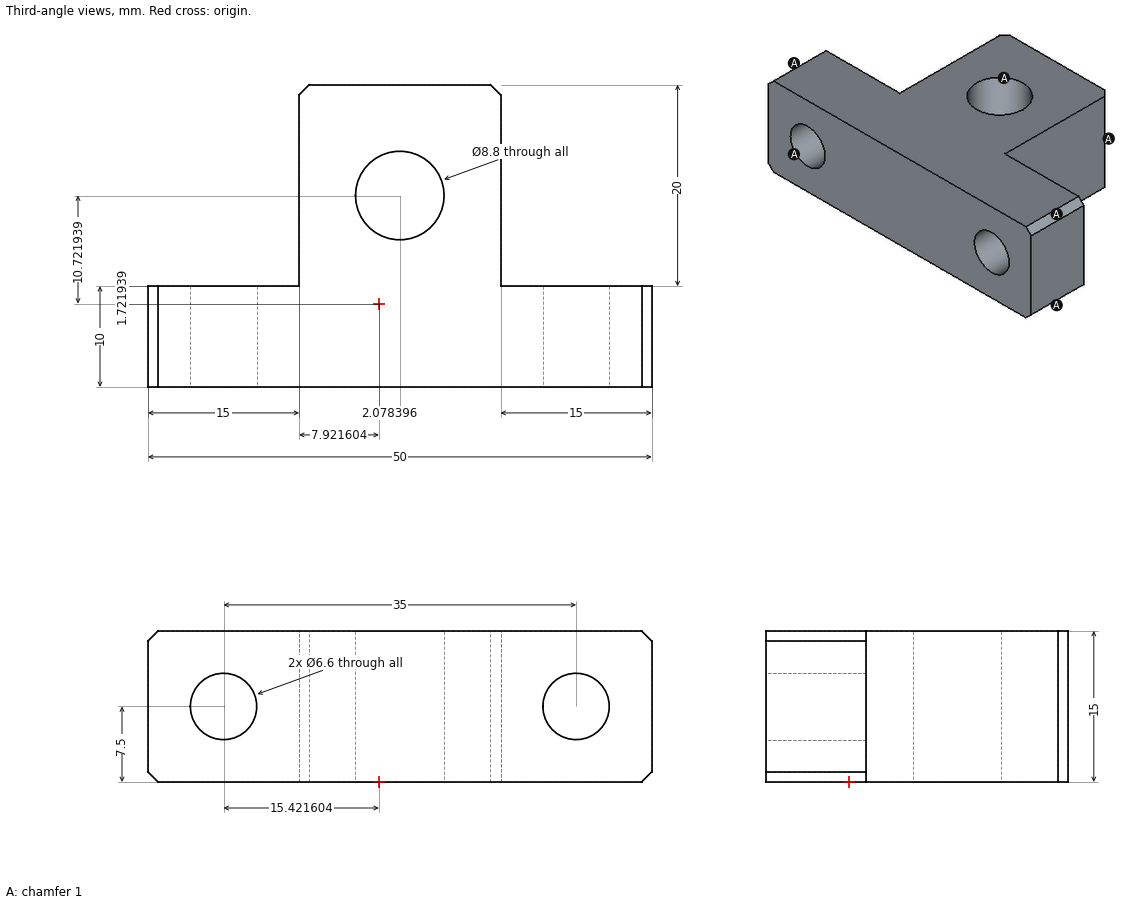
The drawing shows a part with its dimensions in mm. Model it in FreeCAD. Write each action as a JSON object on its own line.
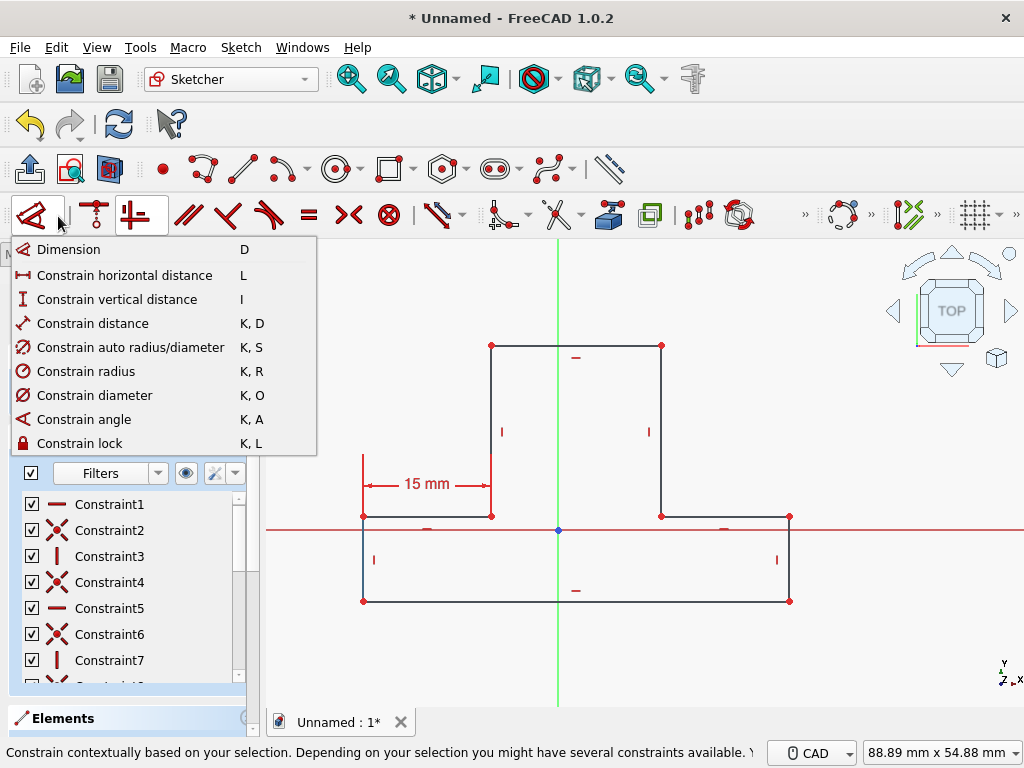
{"action": "left_click", "coordinate": [164, 299]}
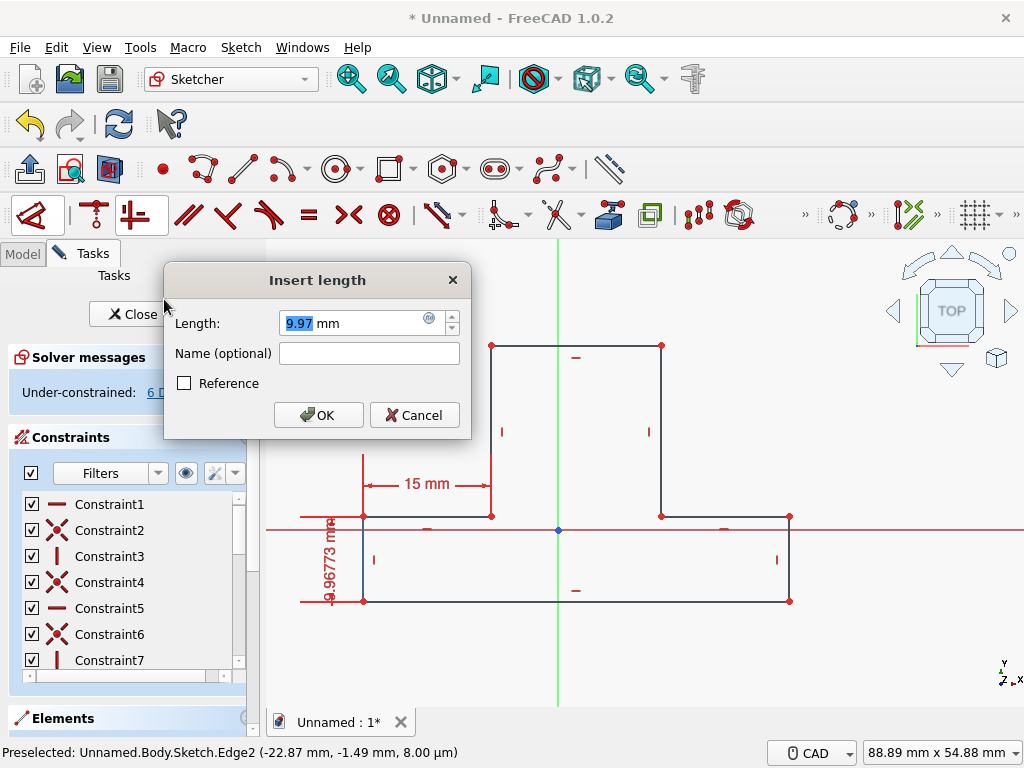
{"action": "type", "text": "10"}
{"action": "key", "text": "Return"}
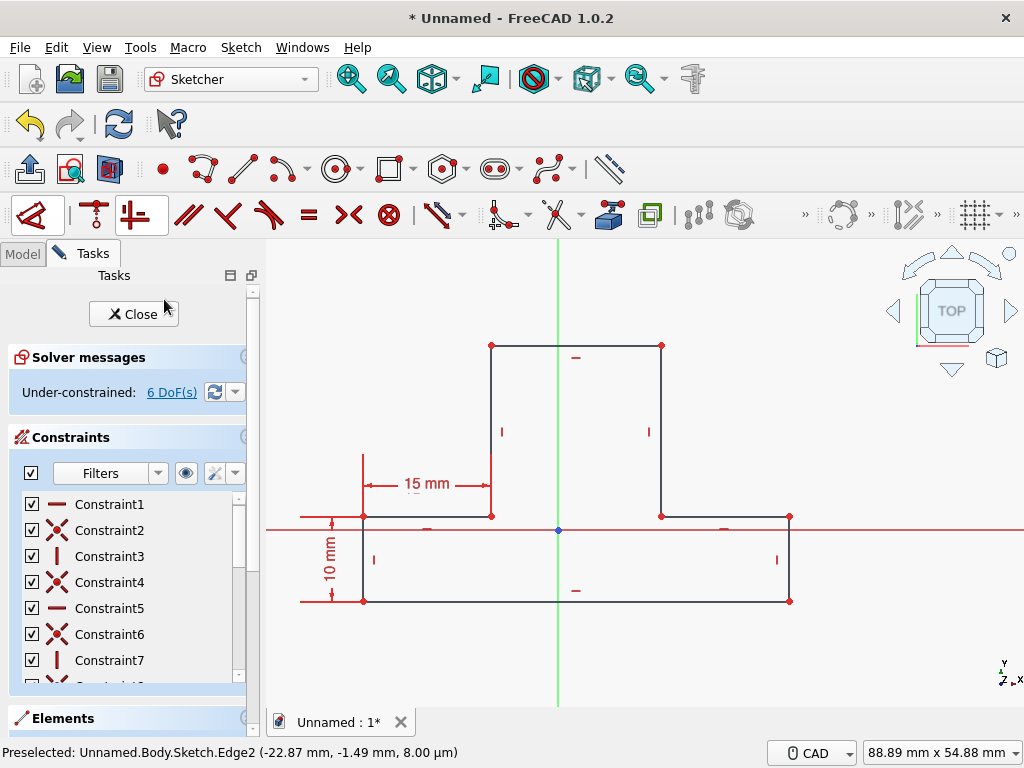
{"action": "left_click", "coordinate": [491, 602]}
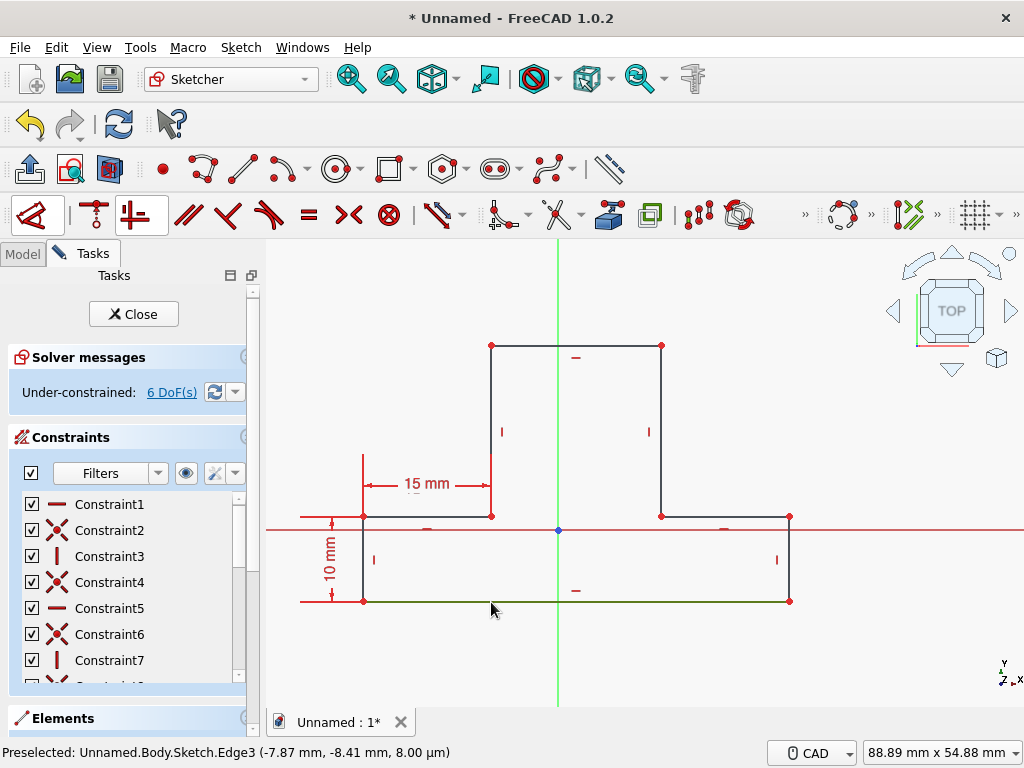
{"action": "left_click", "coordinate": [58, 216]}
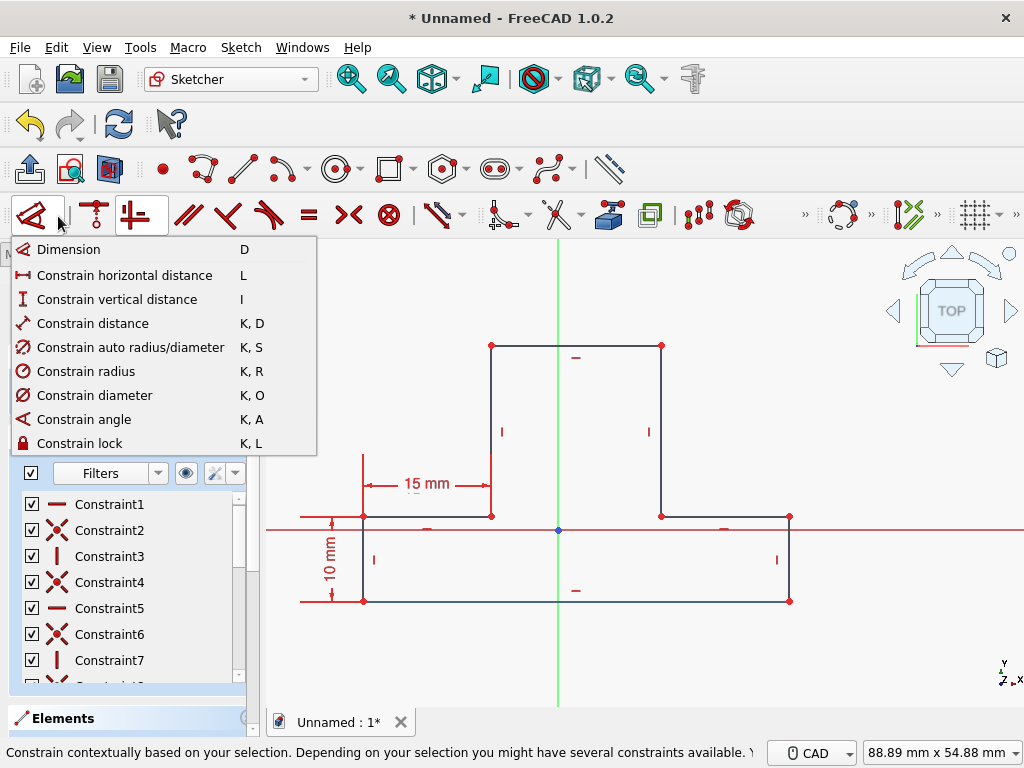
{"action": "left_click", "coordinate": [164, 275]}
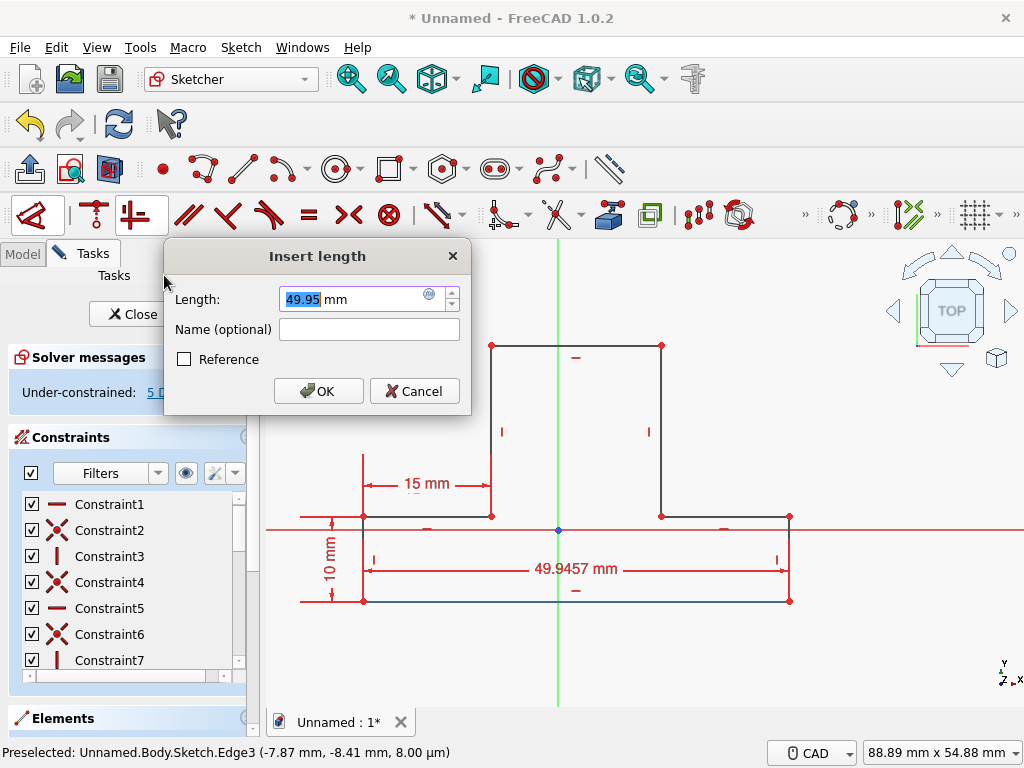
{"action": "type", "text": "50"}
{"action": "key", "text": "Return"}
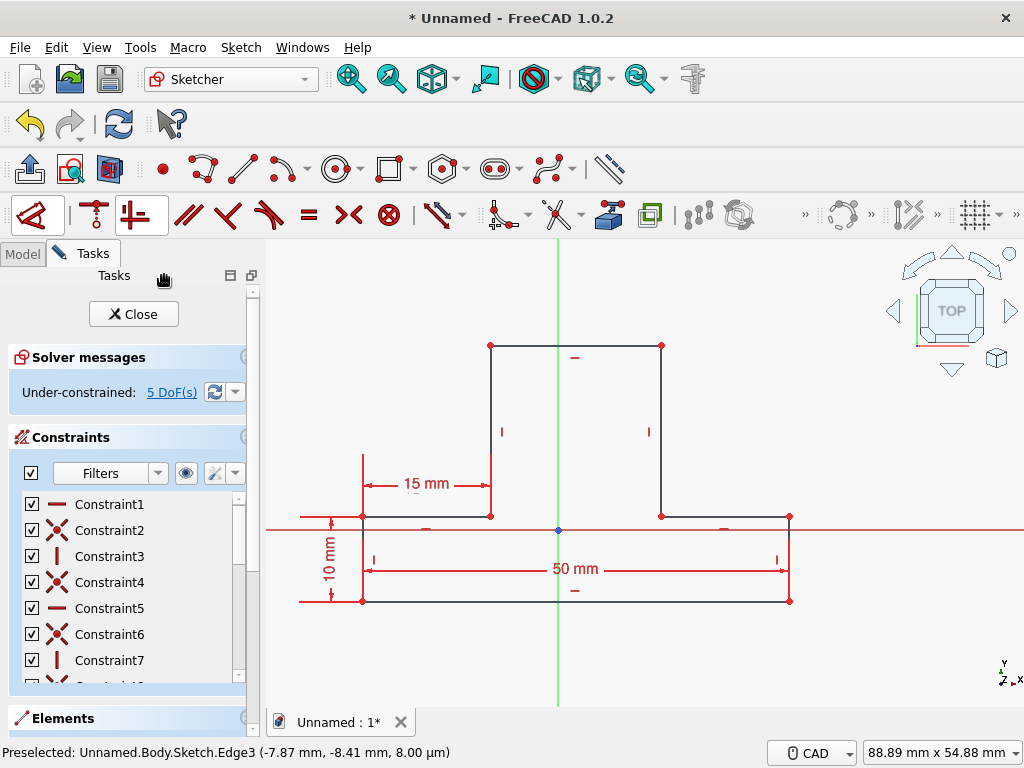
{"action": "left_click", "coordinate": [789, 576]}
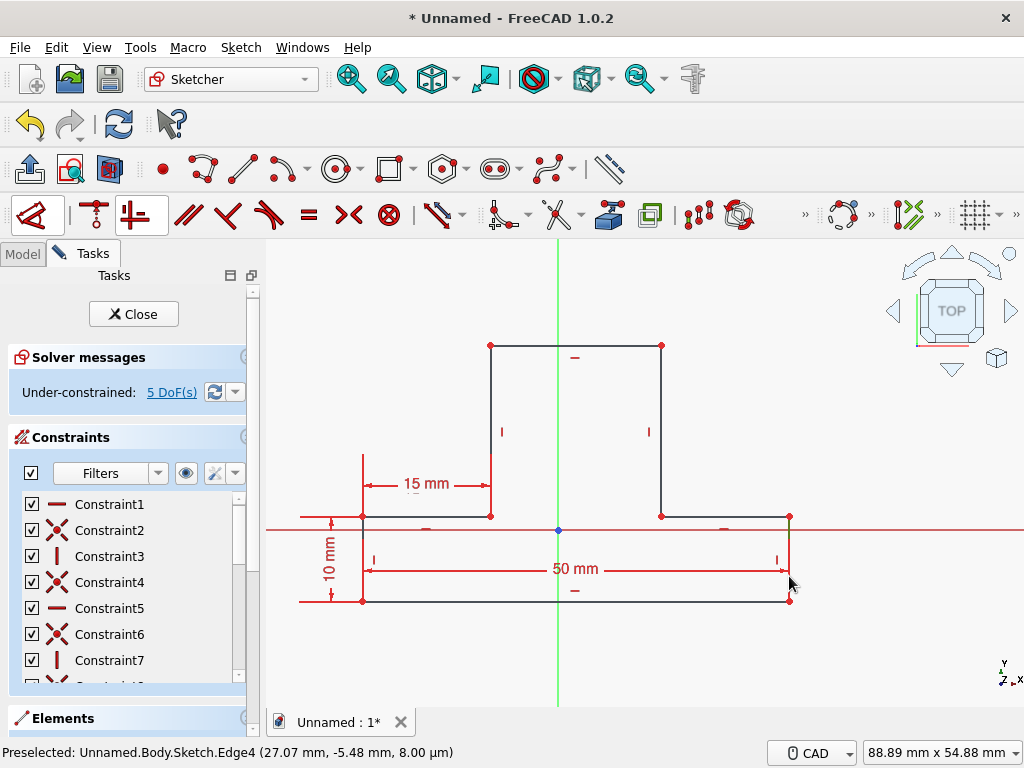
{"action": "key", "text": "i"}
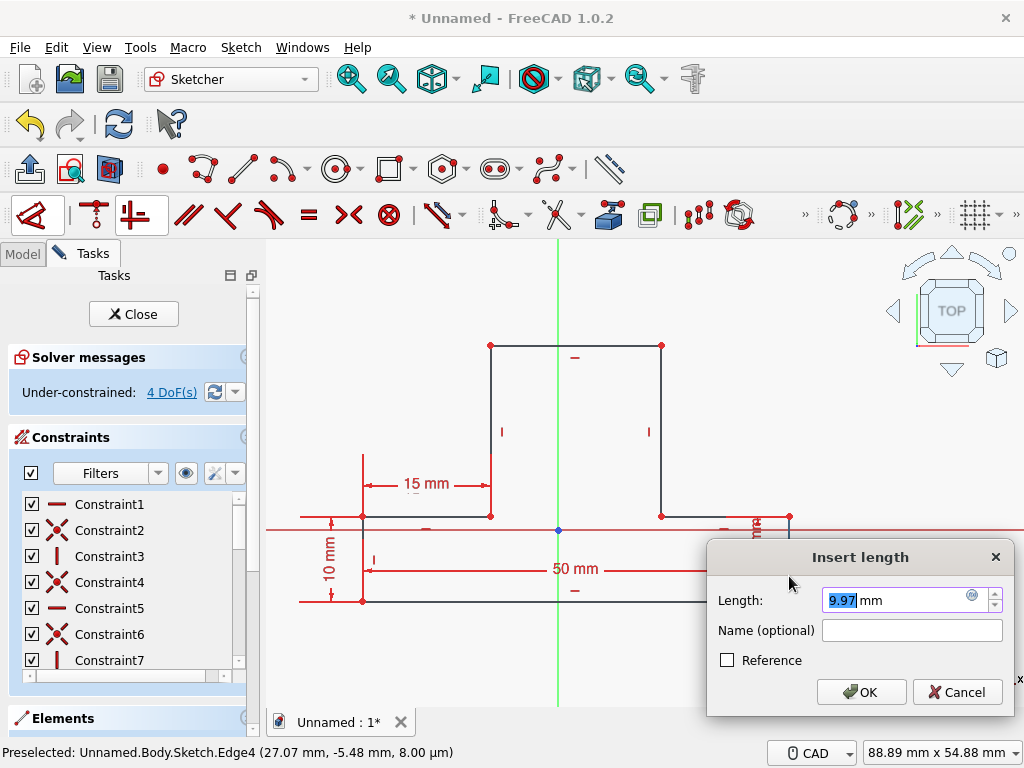
{"action": "type", "text": "10"}
{"action": "key", "text": "Return"}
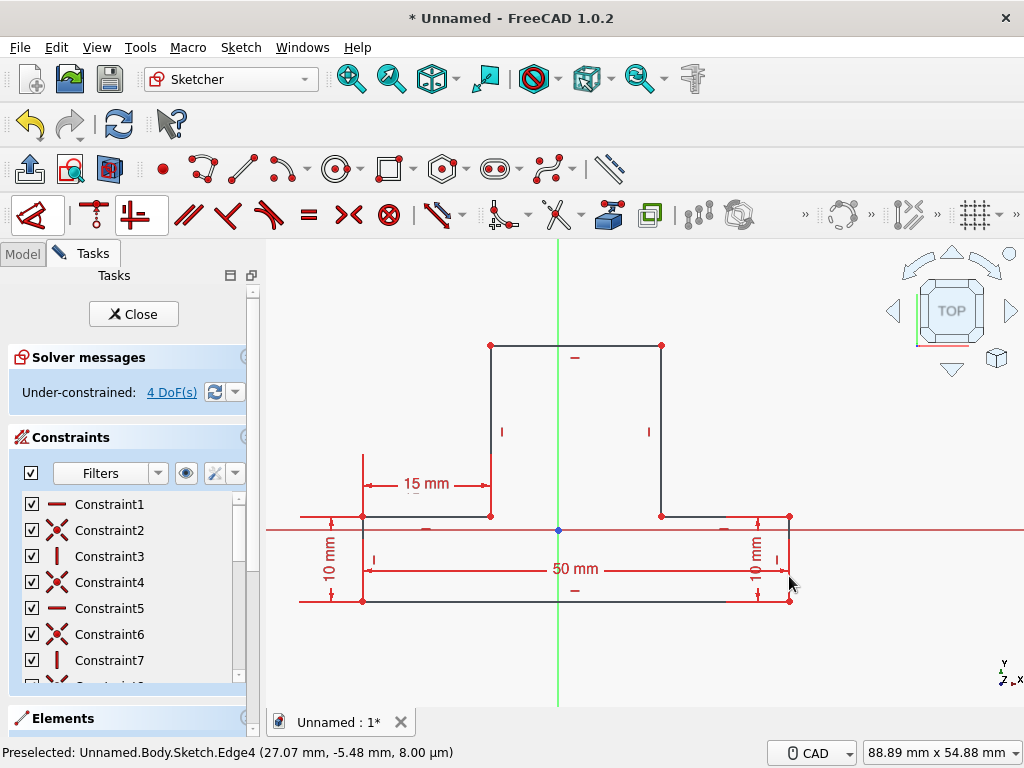
{"action": "left_click", "coordinate": [751, 517]}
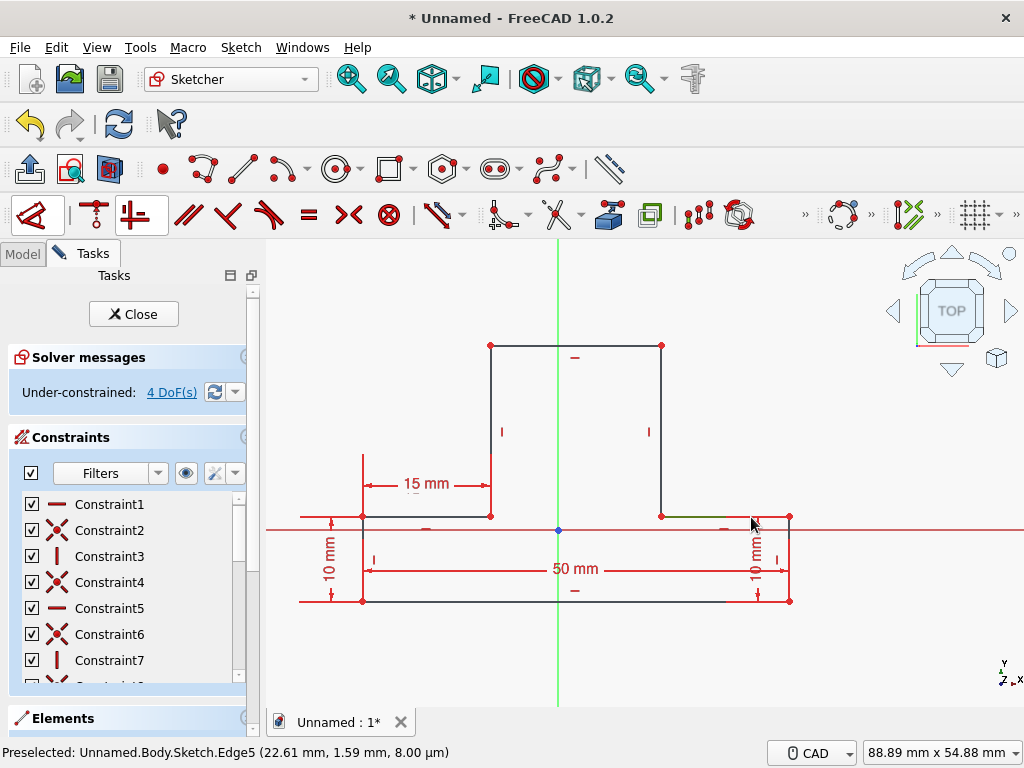
{"action": "key", "text": "l"}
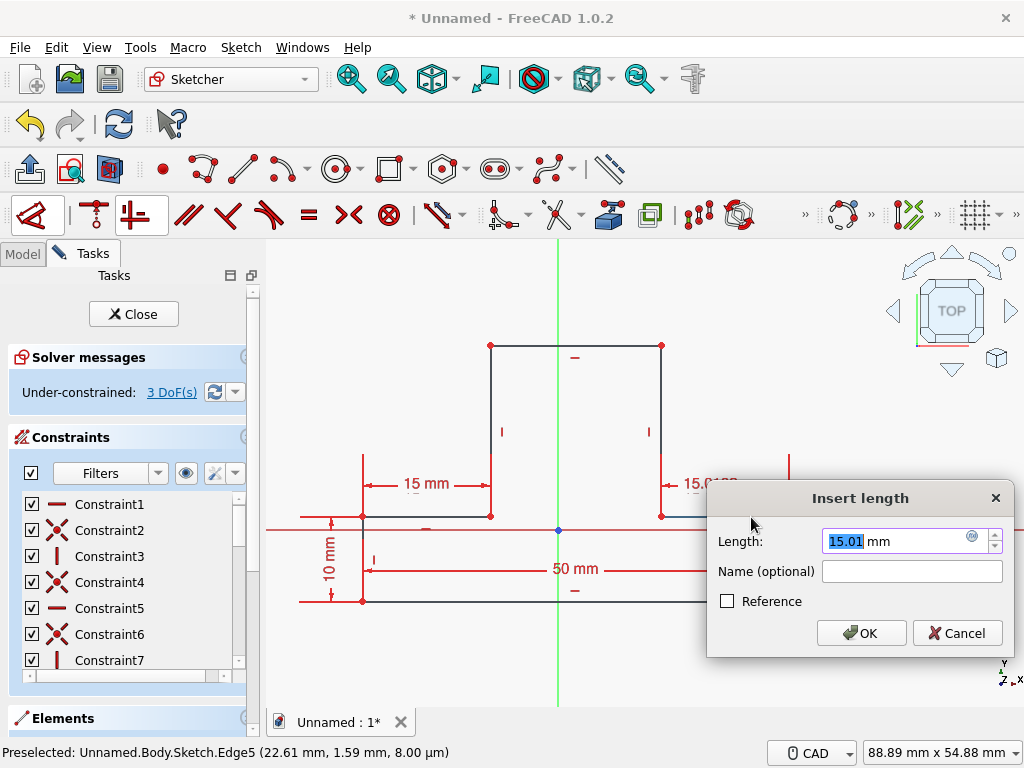
{"action": "type", "text": "15"}
{"action": "key", "text": "Return"}